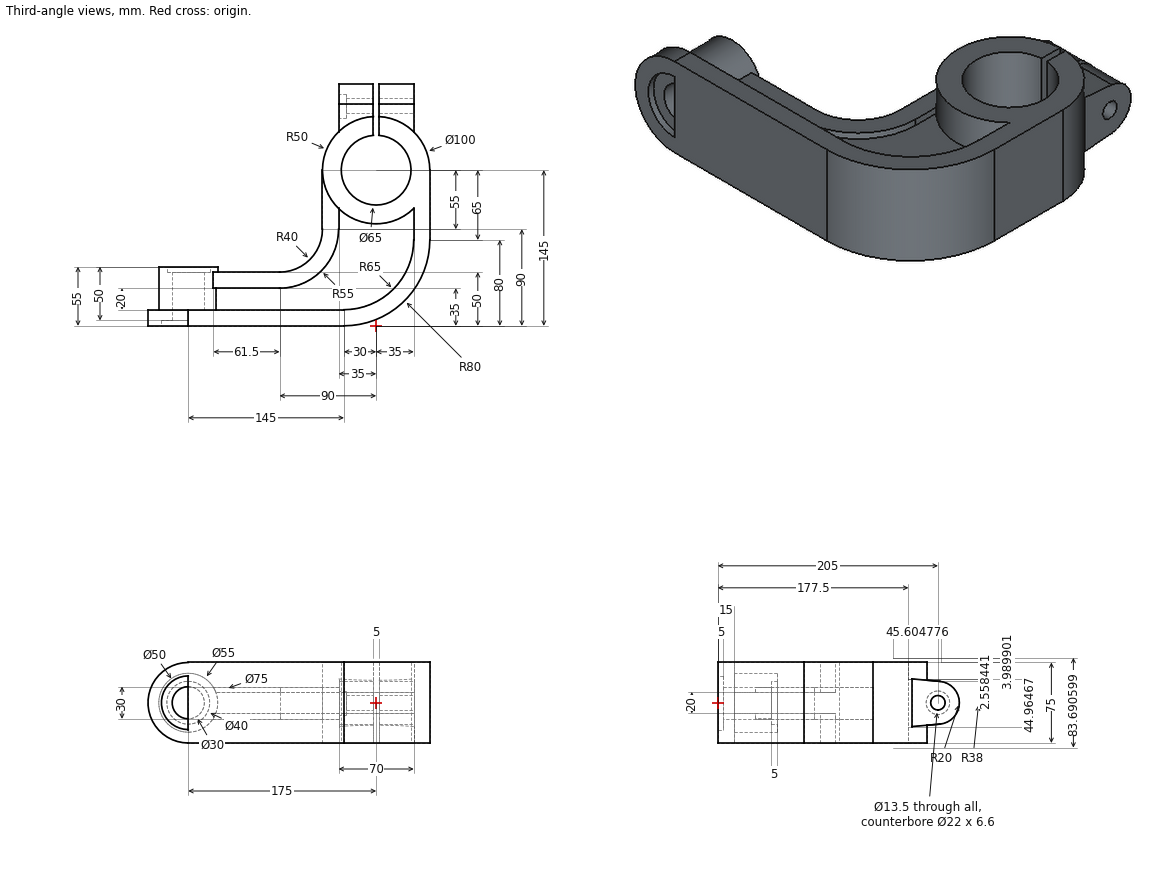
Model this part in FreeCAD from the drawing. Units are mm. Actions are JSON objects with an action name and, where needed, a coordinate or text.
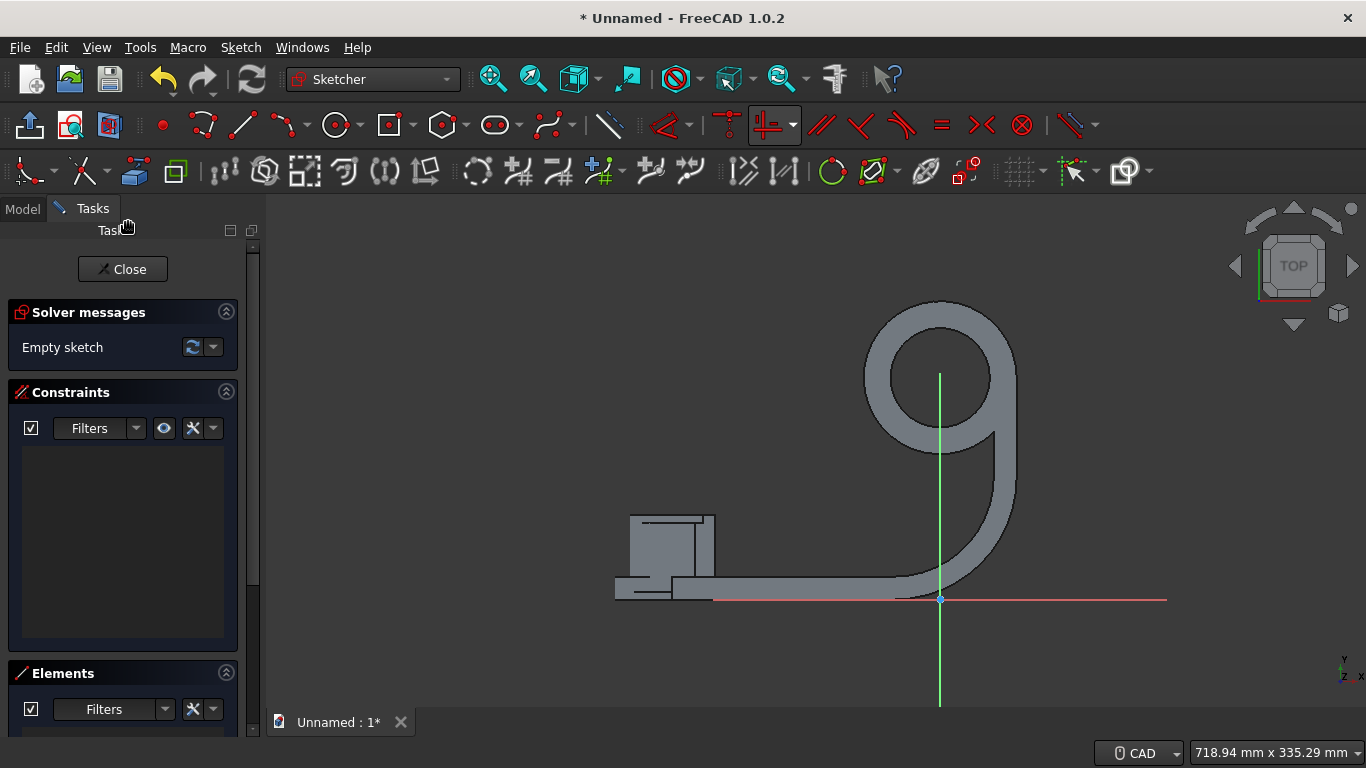
{"action": "scroll", "coordinate": [977, 596], "scroll_direction": "up", "scroll_amount": 3}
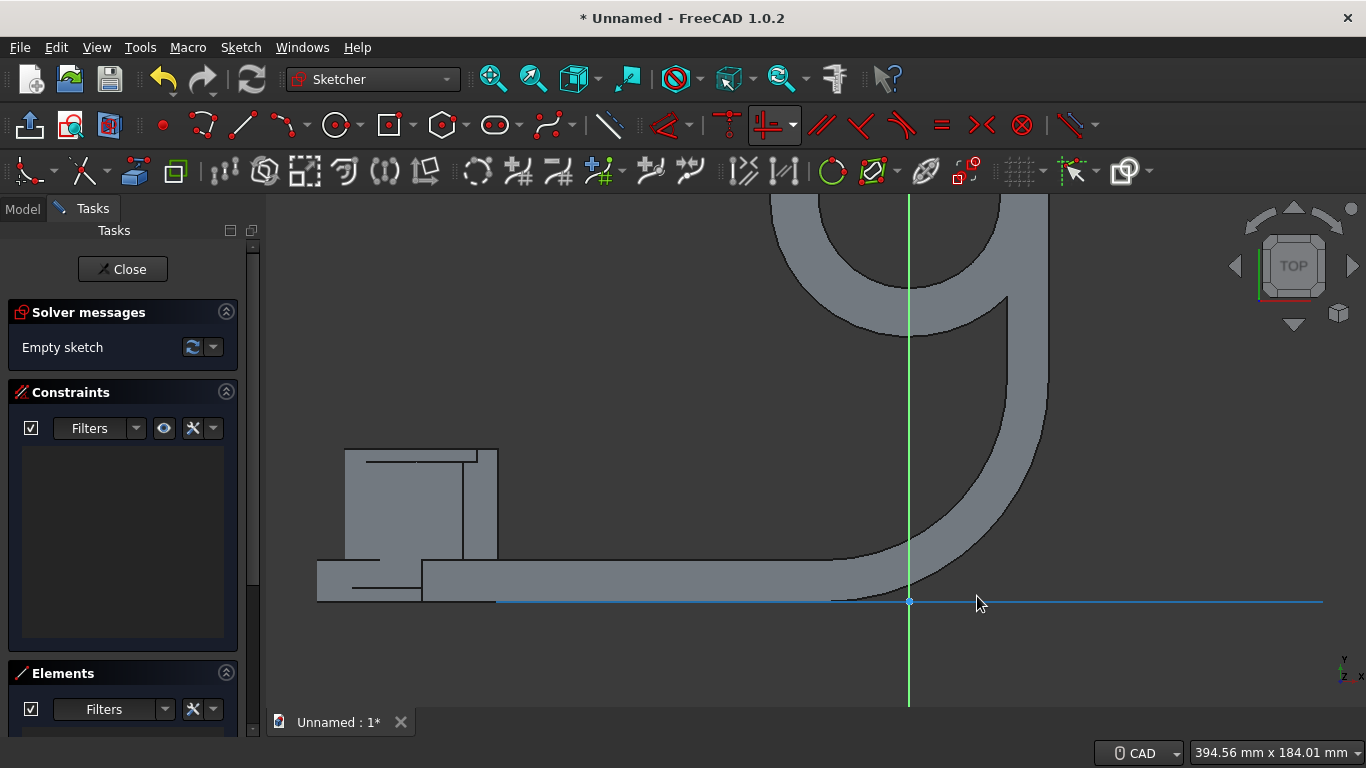
{"action": "key", "text": "g l"}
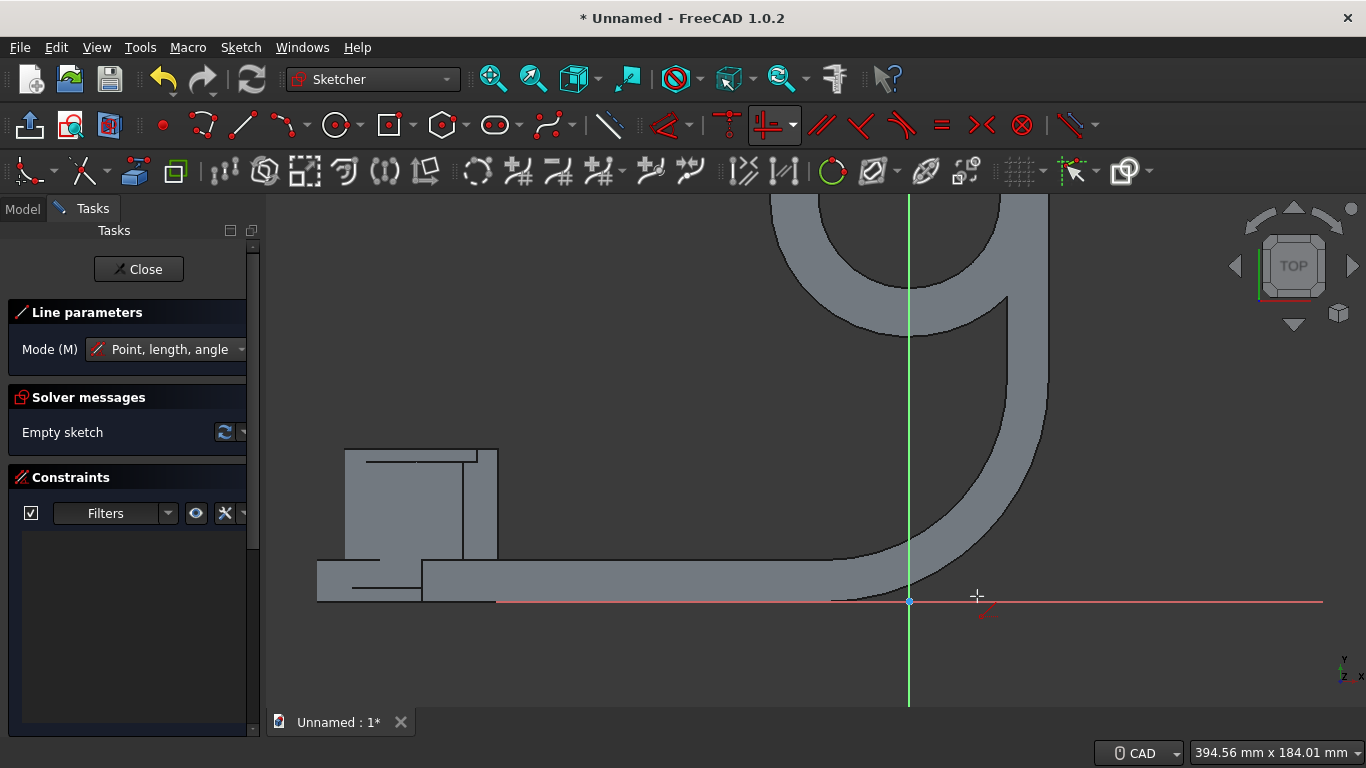
{"action": "left_click", "coordinate": [1007, 379]}
{"action": "left_click", "coordinate": [1007, 297]}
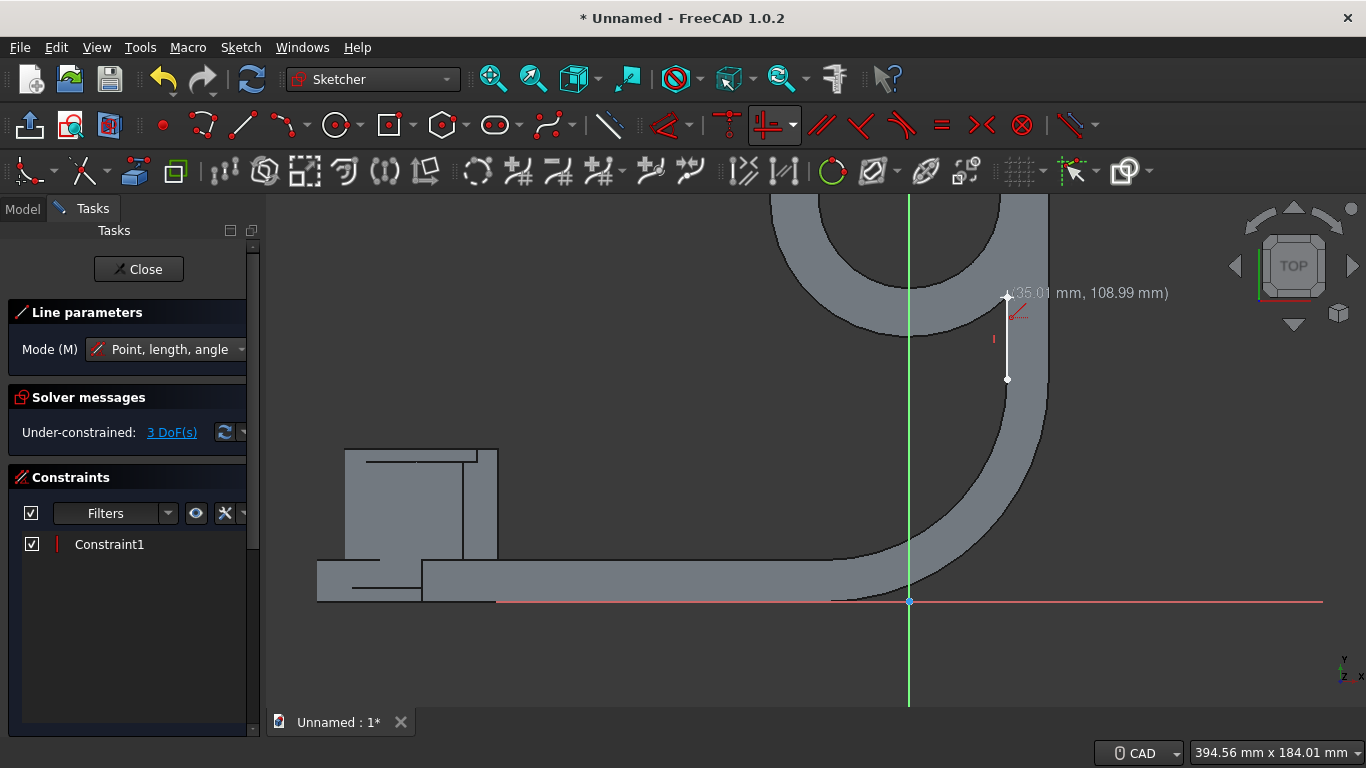
{"action": "left_click", "coordinate": [812, 297]}
{"action": "left_click", "coordinate": [812, 351]}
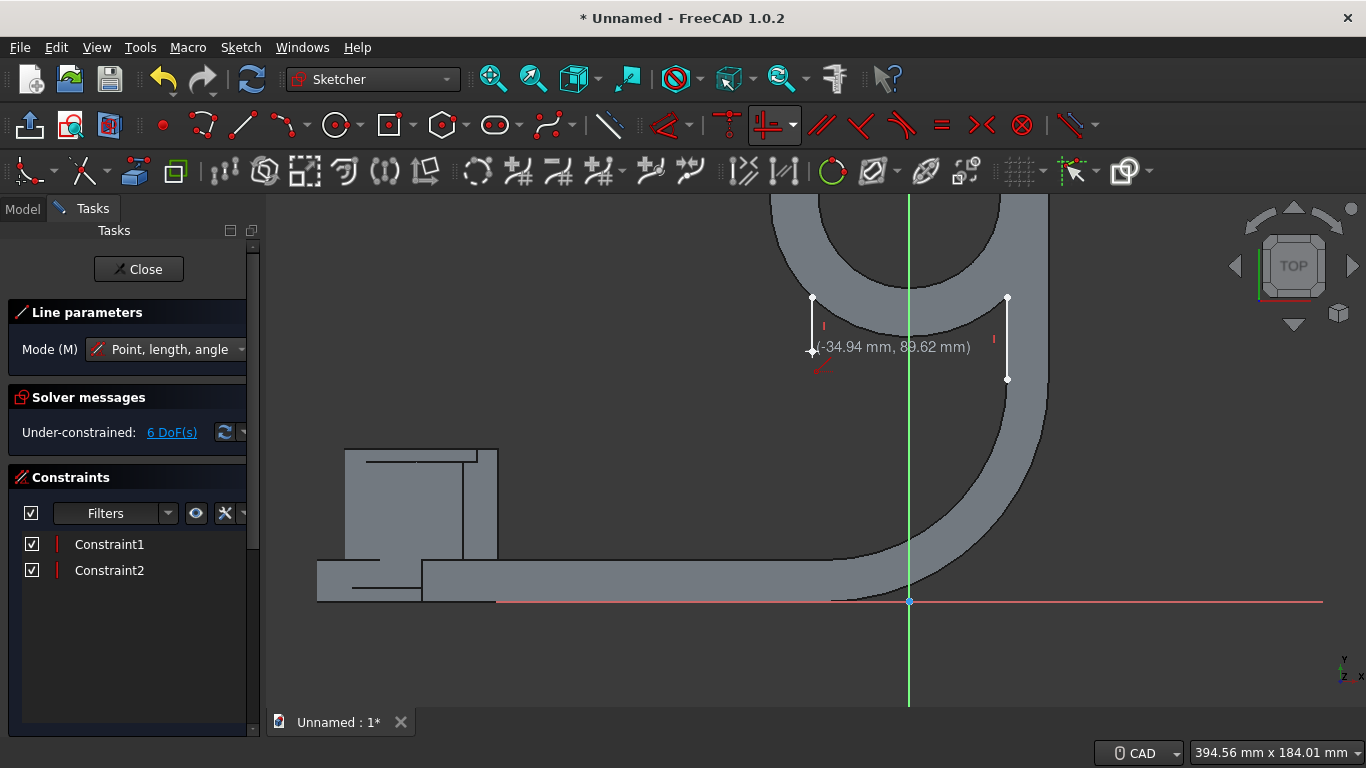
{"action": "key", "text": "g m"}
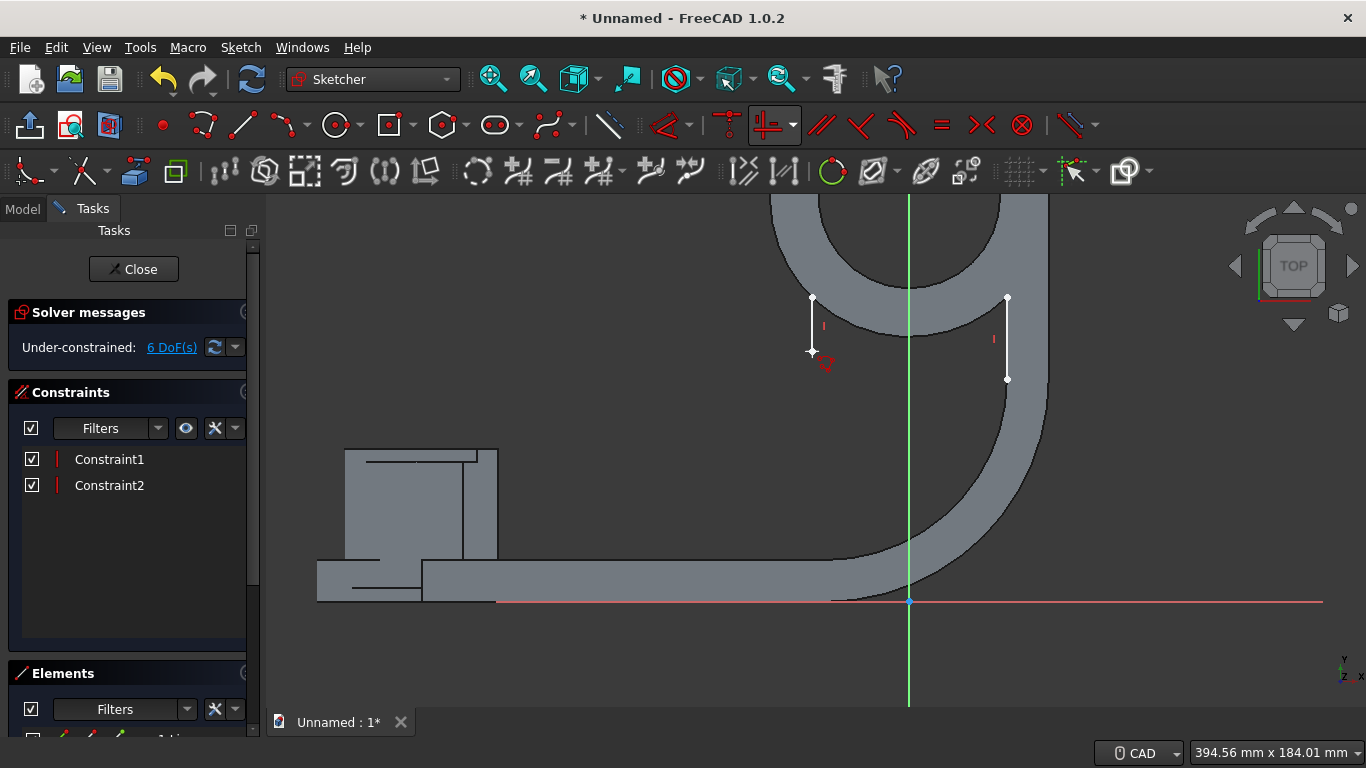
{"action": "left_click", "coordinate": [658, 504]}
{"action": "left_click", "coordinate": [487, 504]}
{"action": "left_click", "coordinate": [487, 560]}
{"action": "left_click", "coordinate": [826, 560]}
{"action": "right_click", "coordinate": [826, 560]}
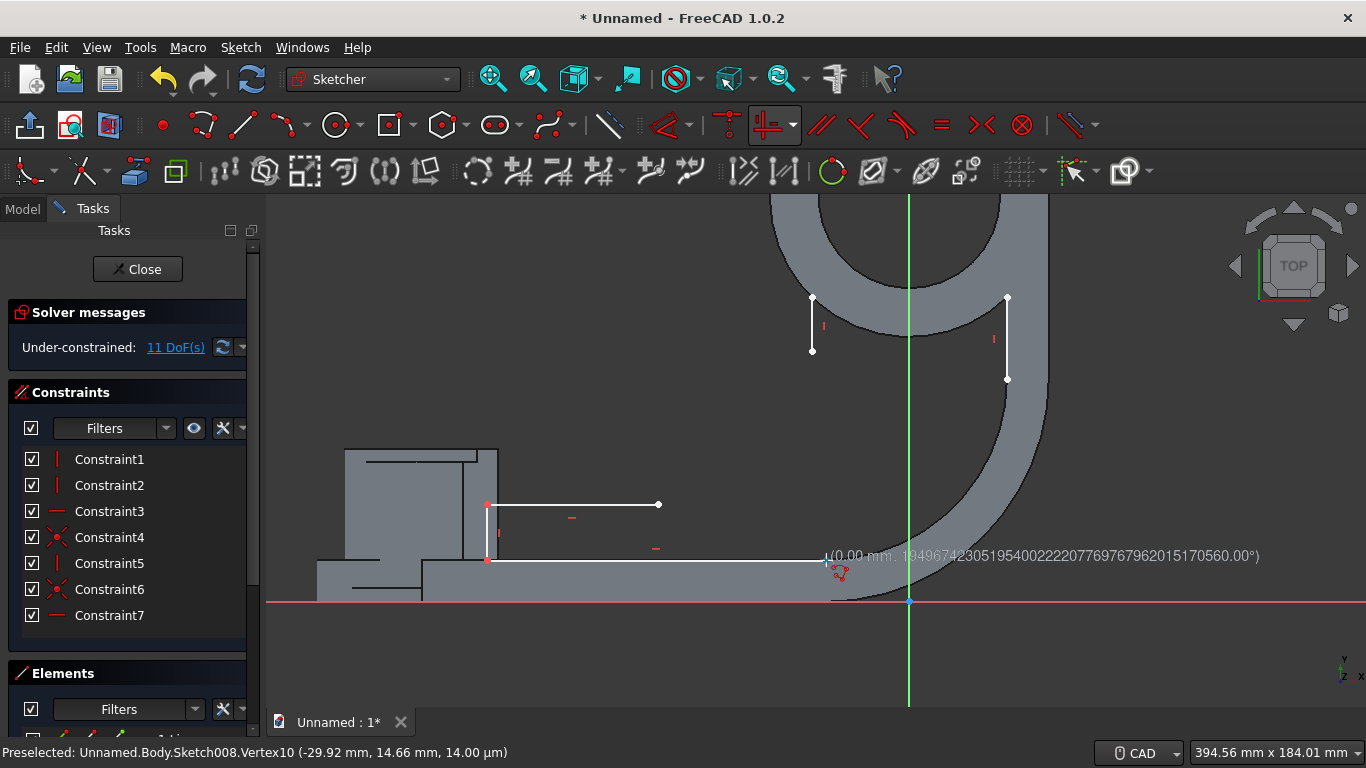
{"action": "key", "text": "g 3 a"}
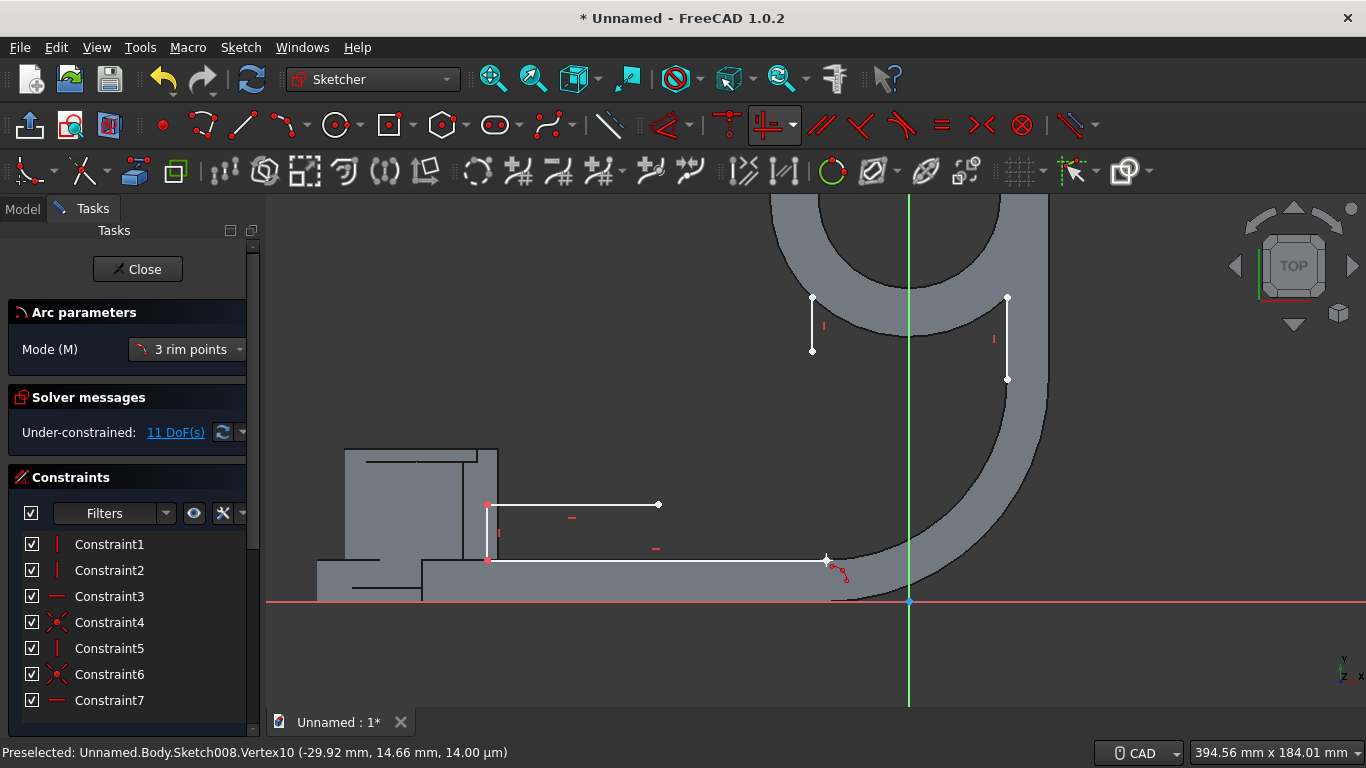
{"action": "left_click", "coordinate": [1007, 298]}
{"action": "left_click", "coordinate": [812, 298]}
{"action": "left_click", "coordinate": [888, 335]}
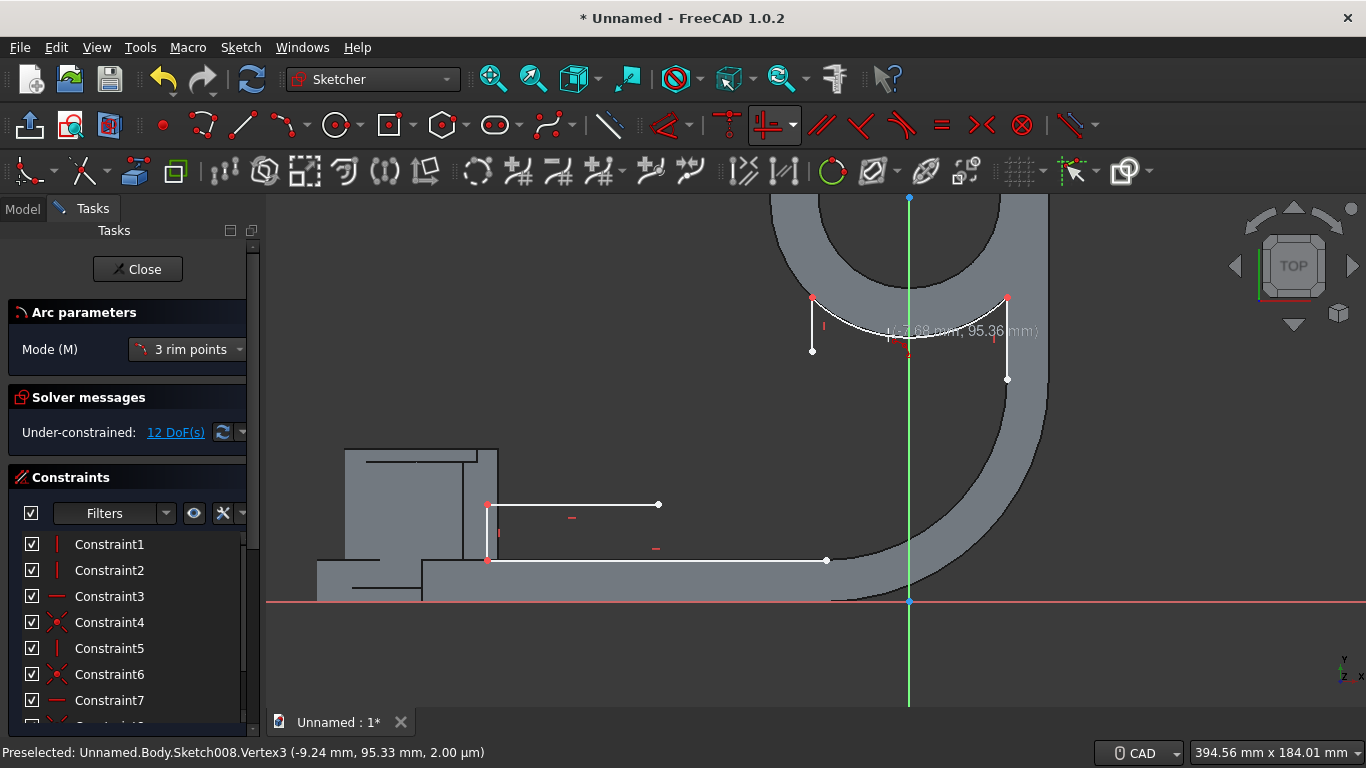
{"action": "left_click", "coordinate": [812, 352]}
{"action": "left_click", "coordinate": [658, 505]}
{"action": "left_click", "coordinate": [767, 459]}